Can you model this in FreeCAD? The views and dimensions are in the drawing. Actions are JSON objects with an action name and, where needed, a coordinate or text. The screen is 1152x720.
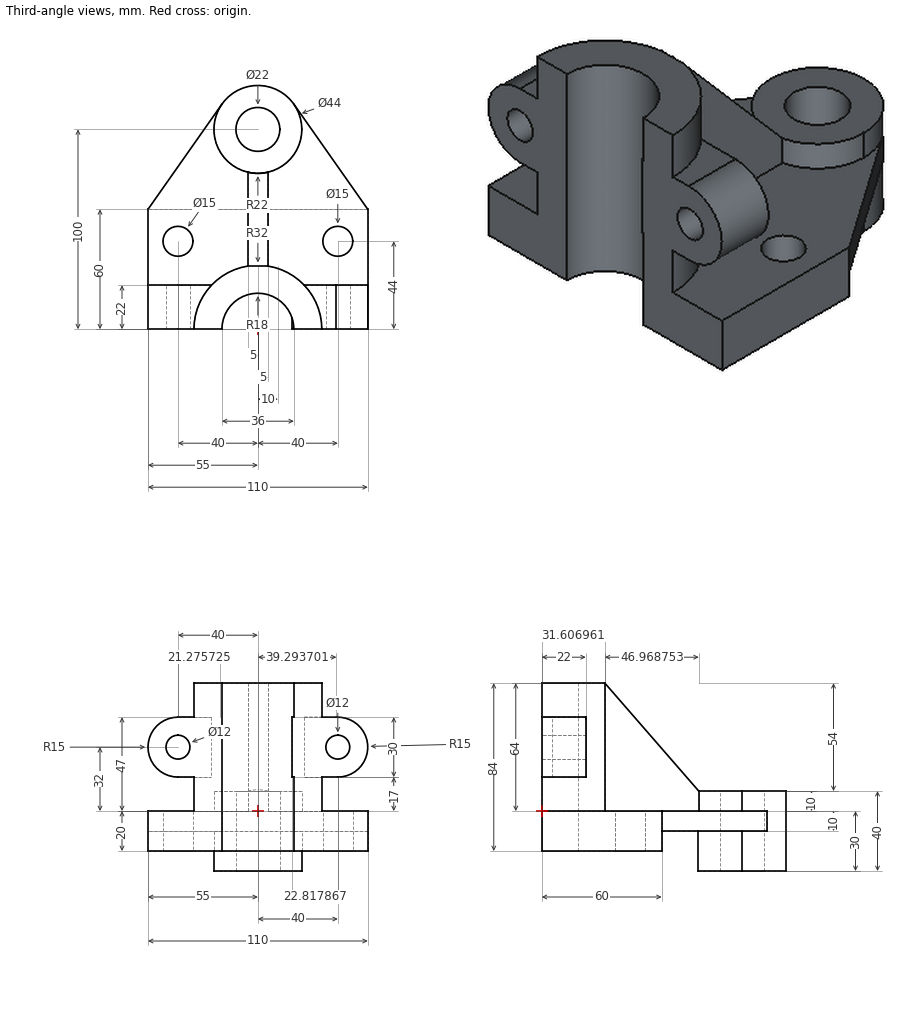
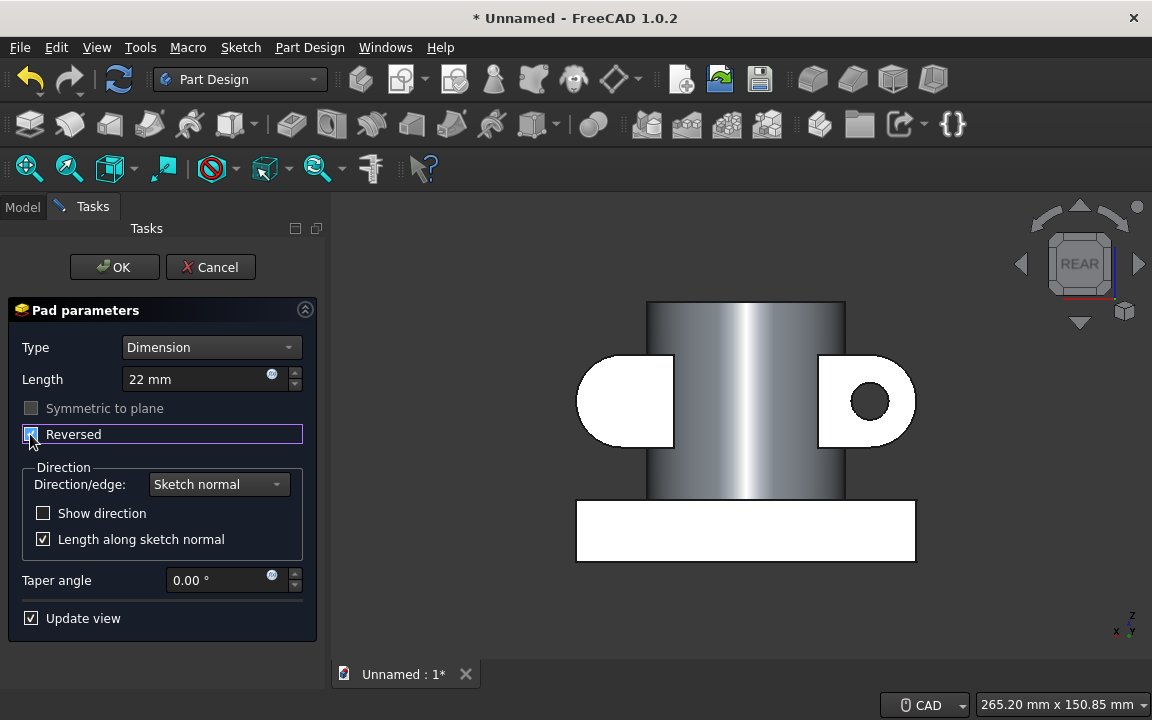
{"action": "left_click", "coordinate": [115, 267]}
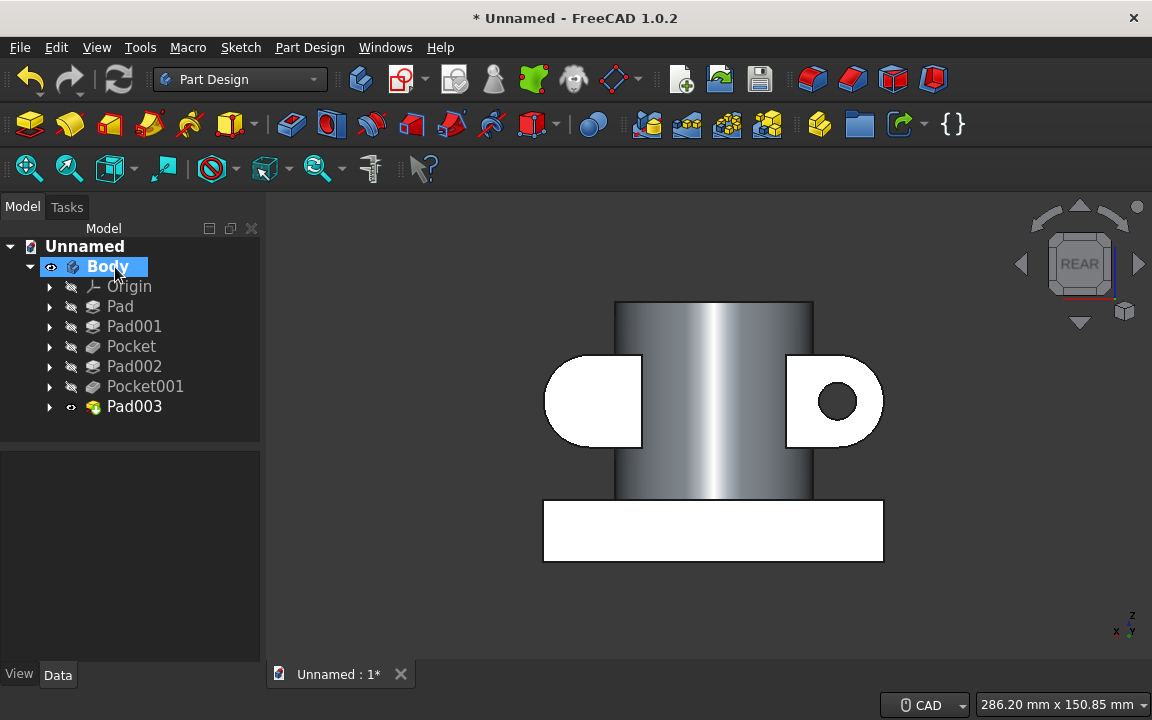
{"action": "left_click", "coordinate": [593, 400]}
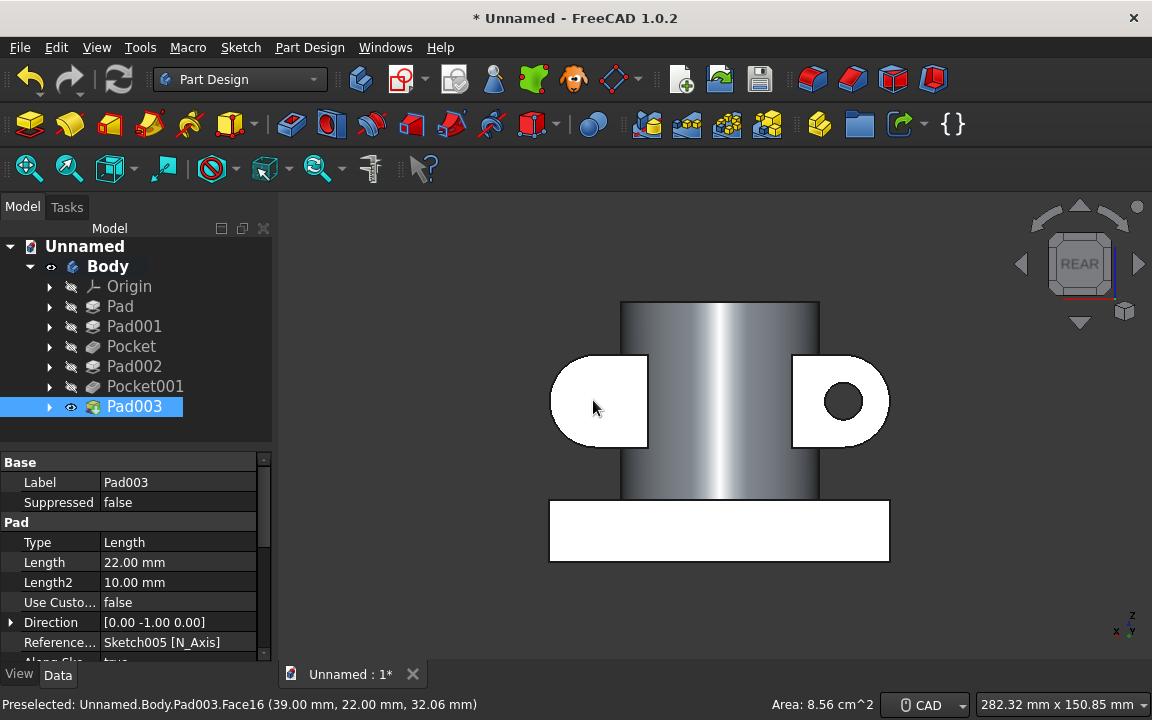
{"action": "left_click", "coordinate": [402, 80]}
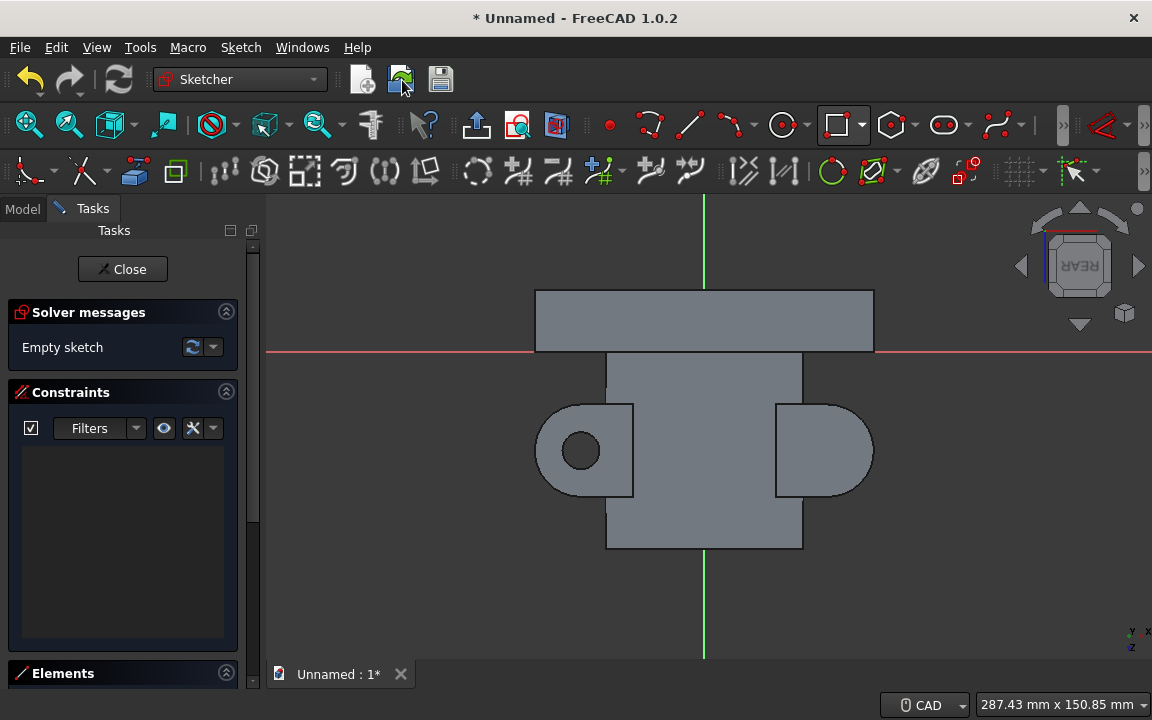
{"action": "left_click", "coordinate": [558, 126]}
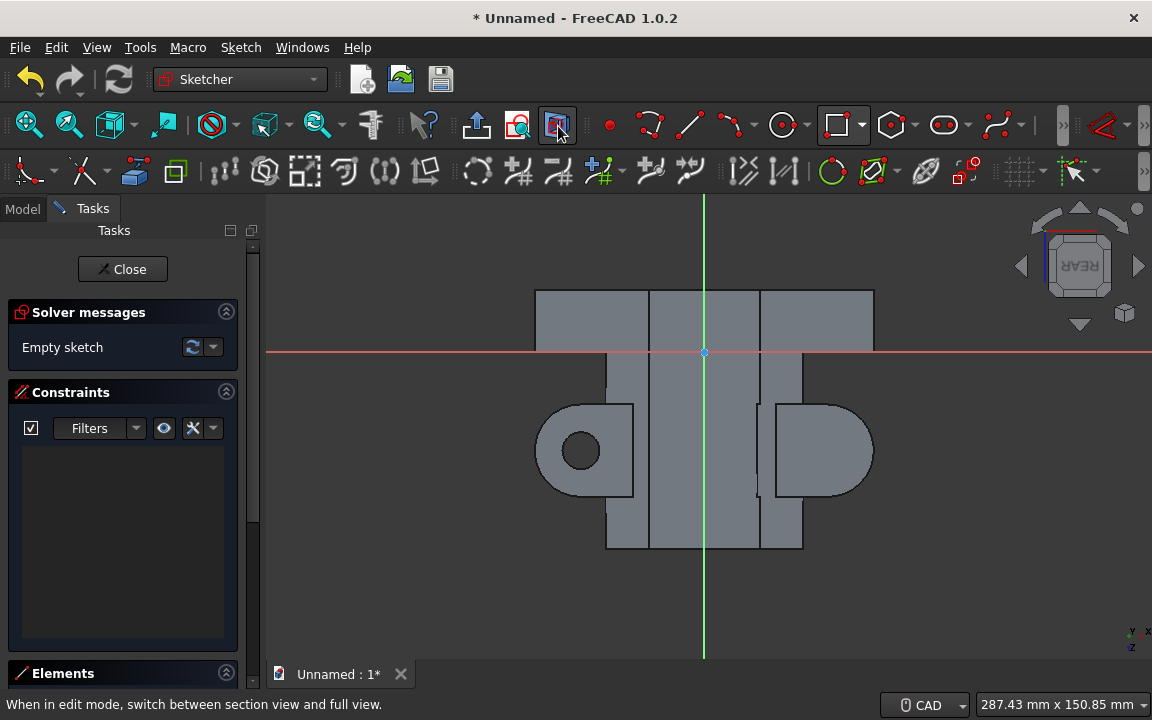
{"action": "scroll", "coordinate": [857, 455], "scroll_direction": "up", "scroll_amount": 10}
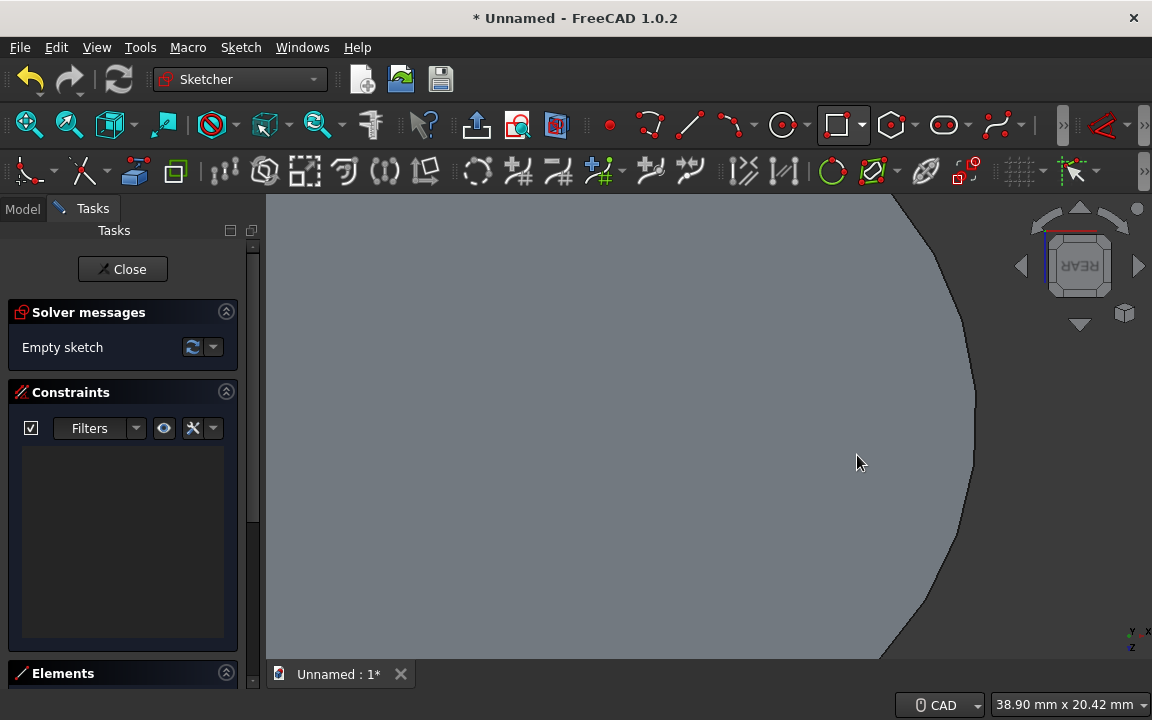
{"action": "left_click", "coordinate": [784, 126]}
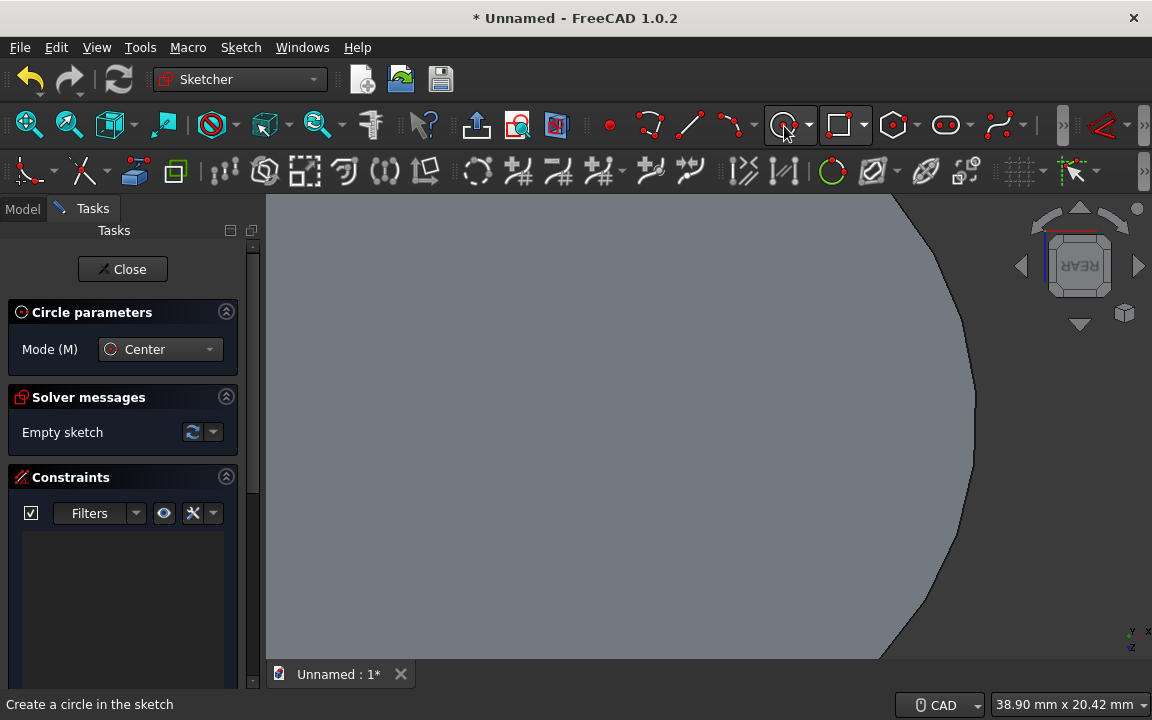
{"action": "left_click", "coordinate": [635, 420]}
{"action": "left_click", "coordinate": [732, 323]}
{"action": "key", "text": "Escape"}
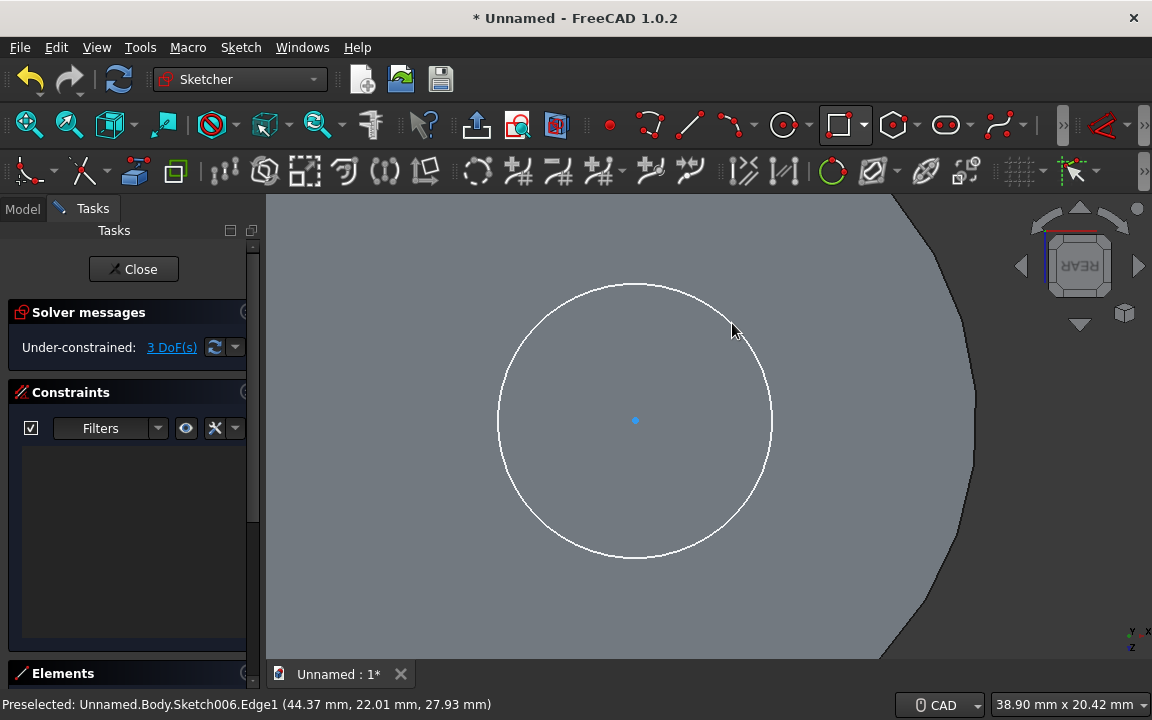
{"action": "left_click", "coordinate": [1102, 126]}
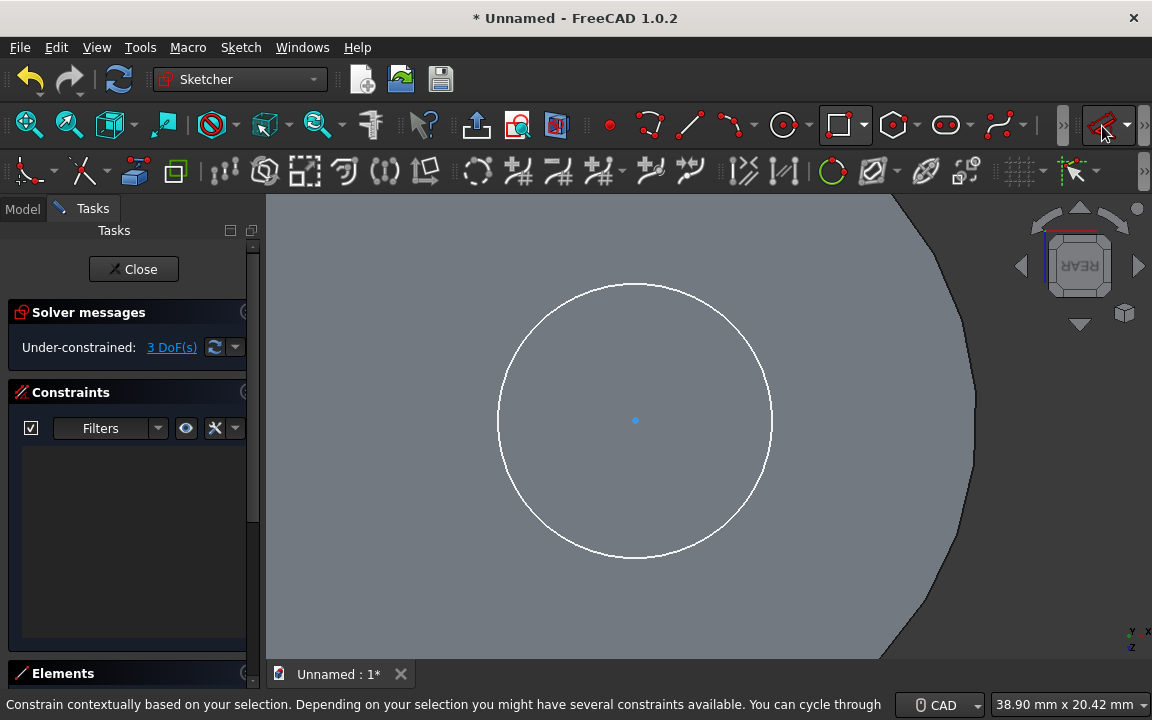
{"action": "left_click", "coordinate": [732, 324]}
{"action": "left_click", "coordinate": [755, 301]}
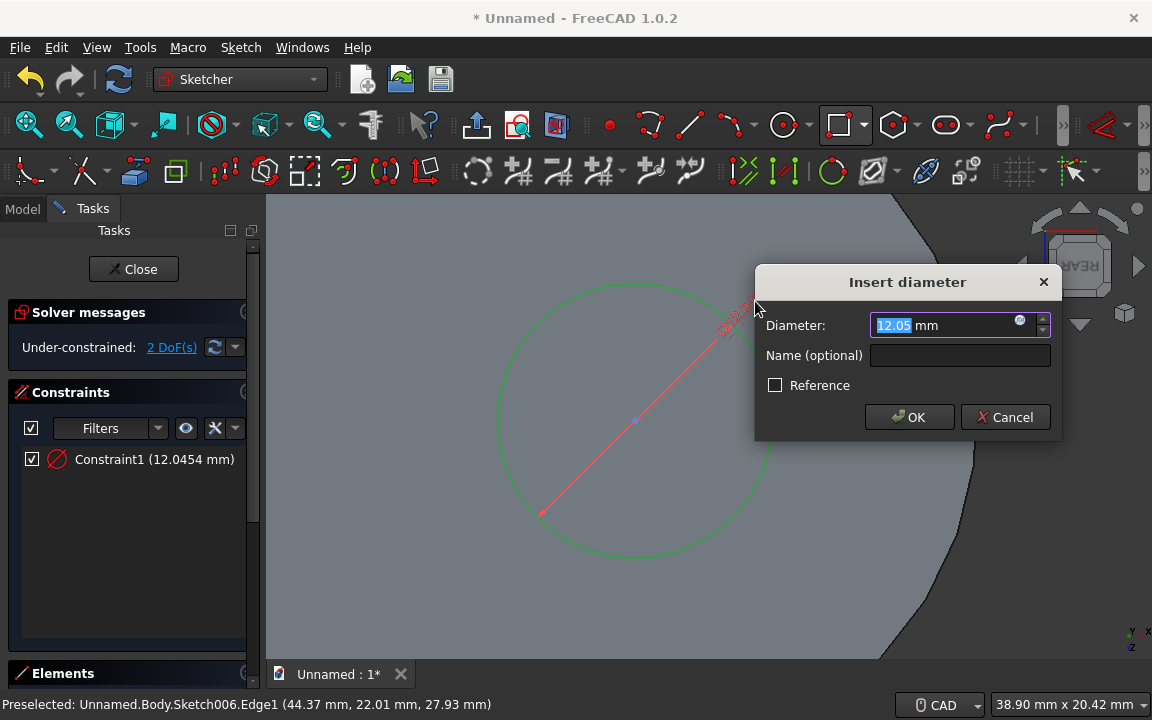
{"action": "type", "text": "12"}
{"action": "key", "text": "Return"}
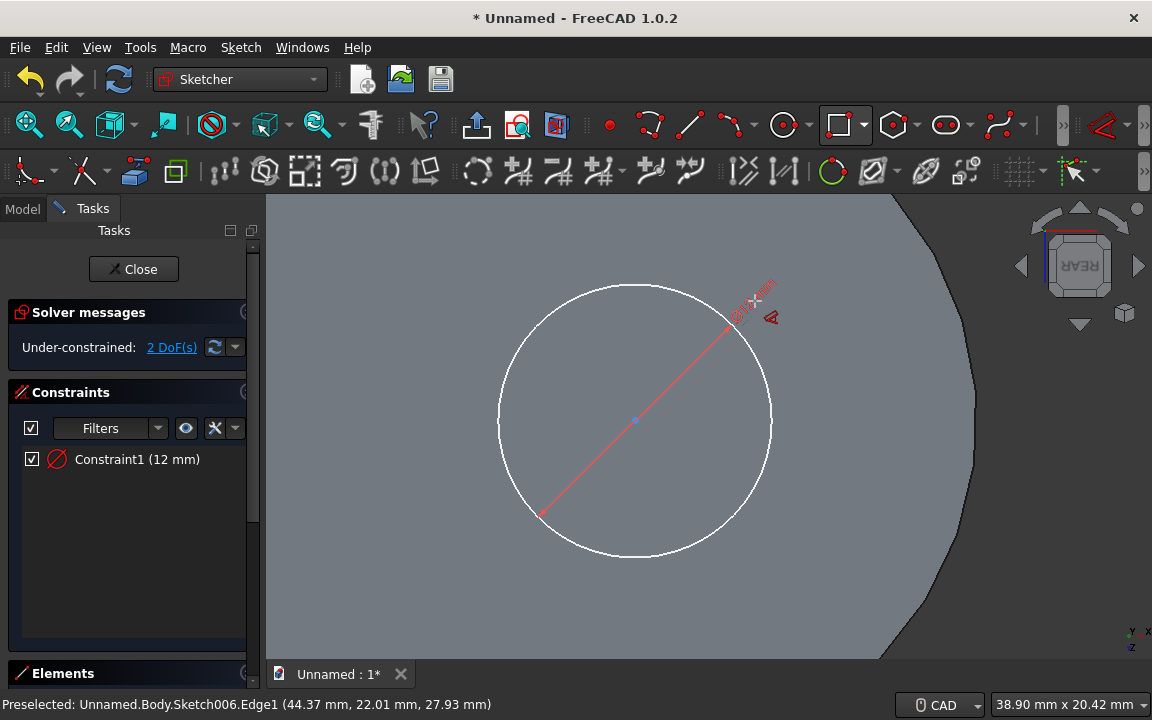
{"action": "left_click", "coordinate": [635, 421]}
{"action": "left_click", "coordinate": [464, 455]}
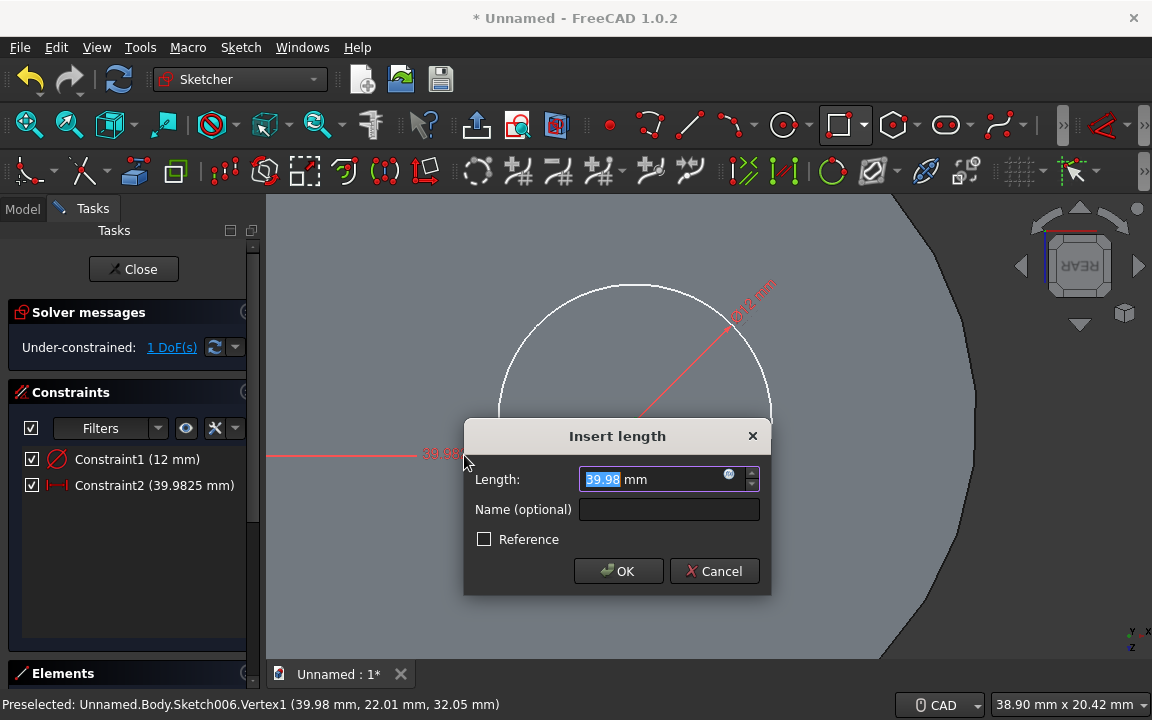
{"action": "type", "text": "40"}
{"action": "key", "text": "Return"}